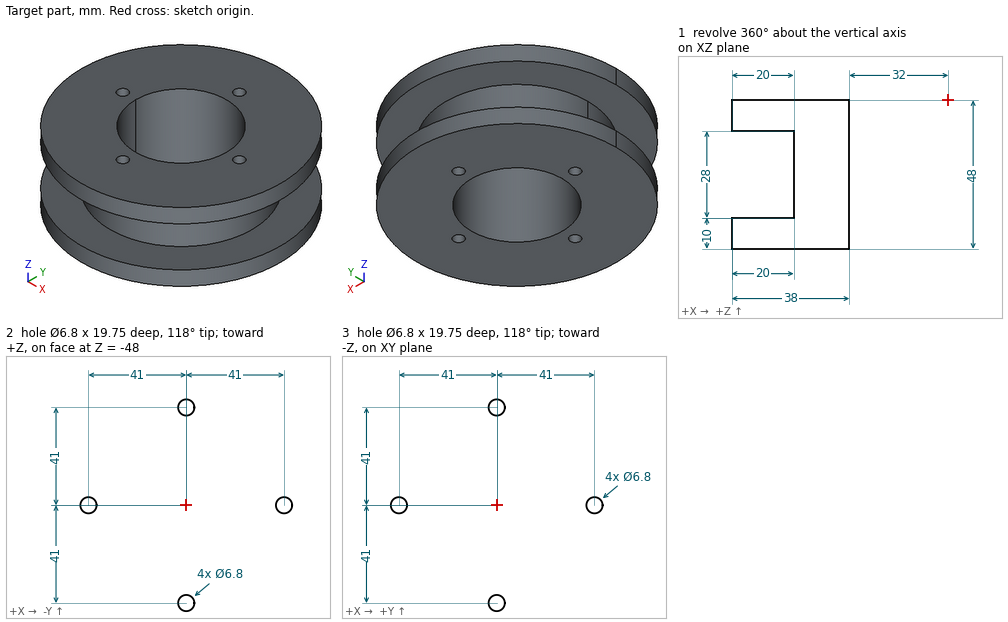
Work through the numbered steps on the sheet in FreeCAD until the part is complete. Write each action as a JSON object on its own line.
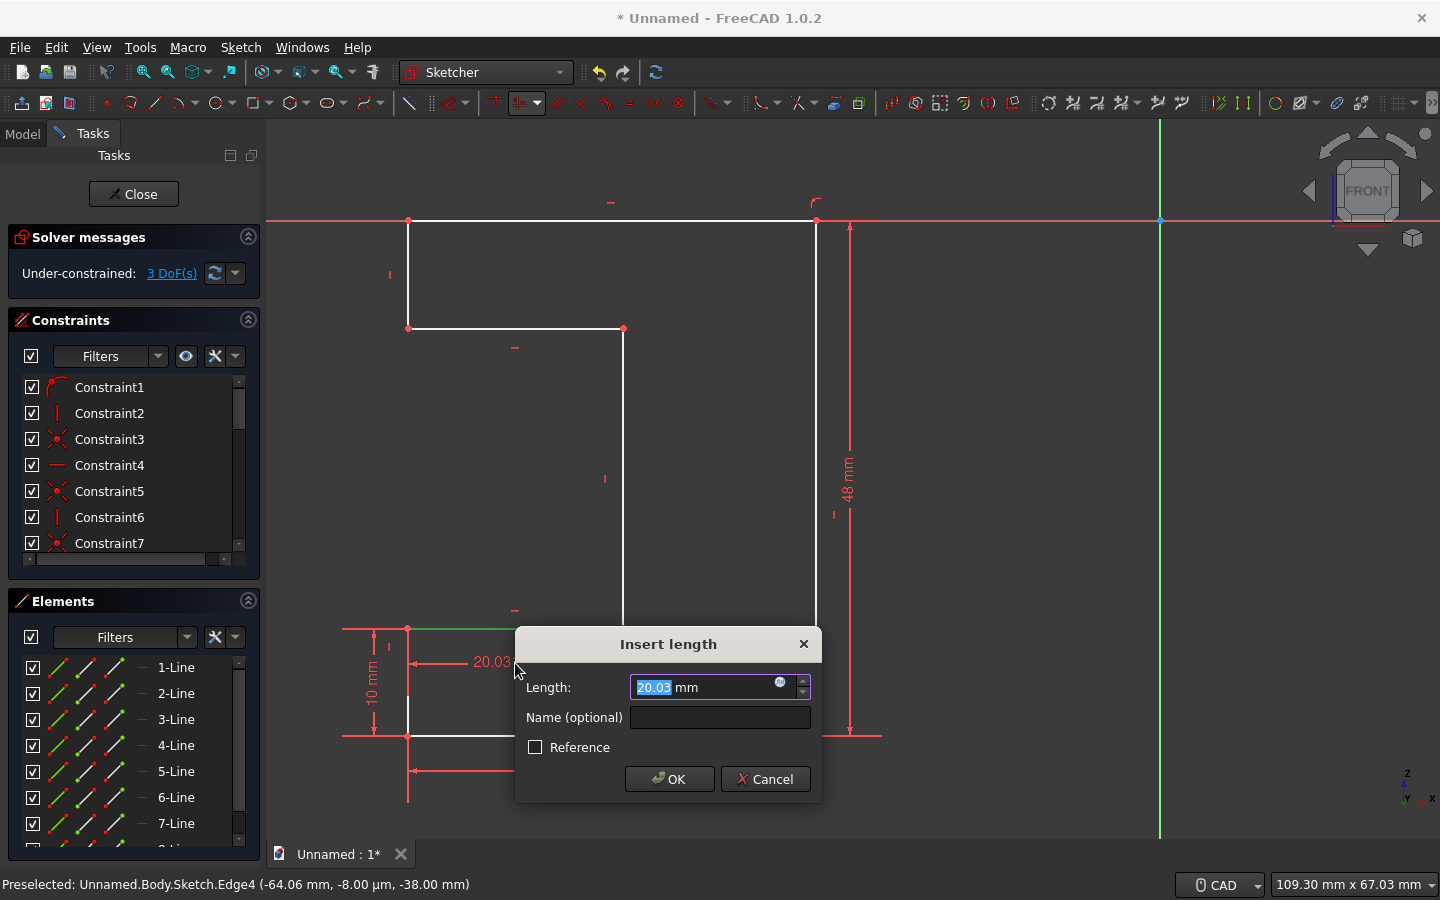
{"action": "type", "text": "20"}
{"action": "key", "text": "Return"}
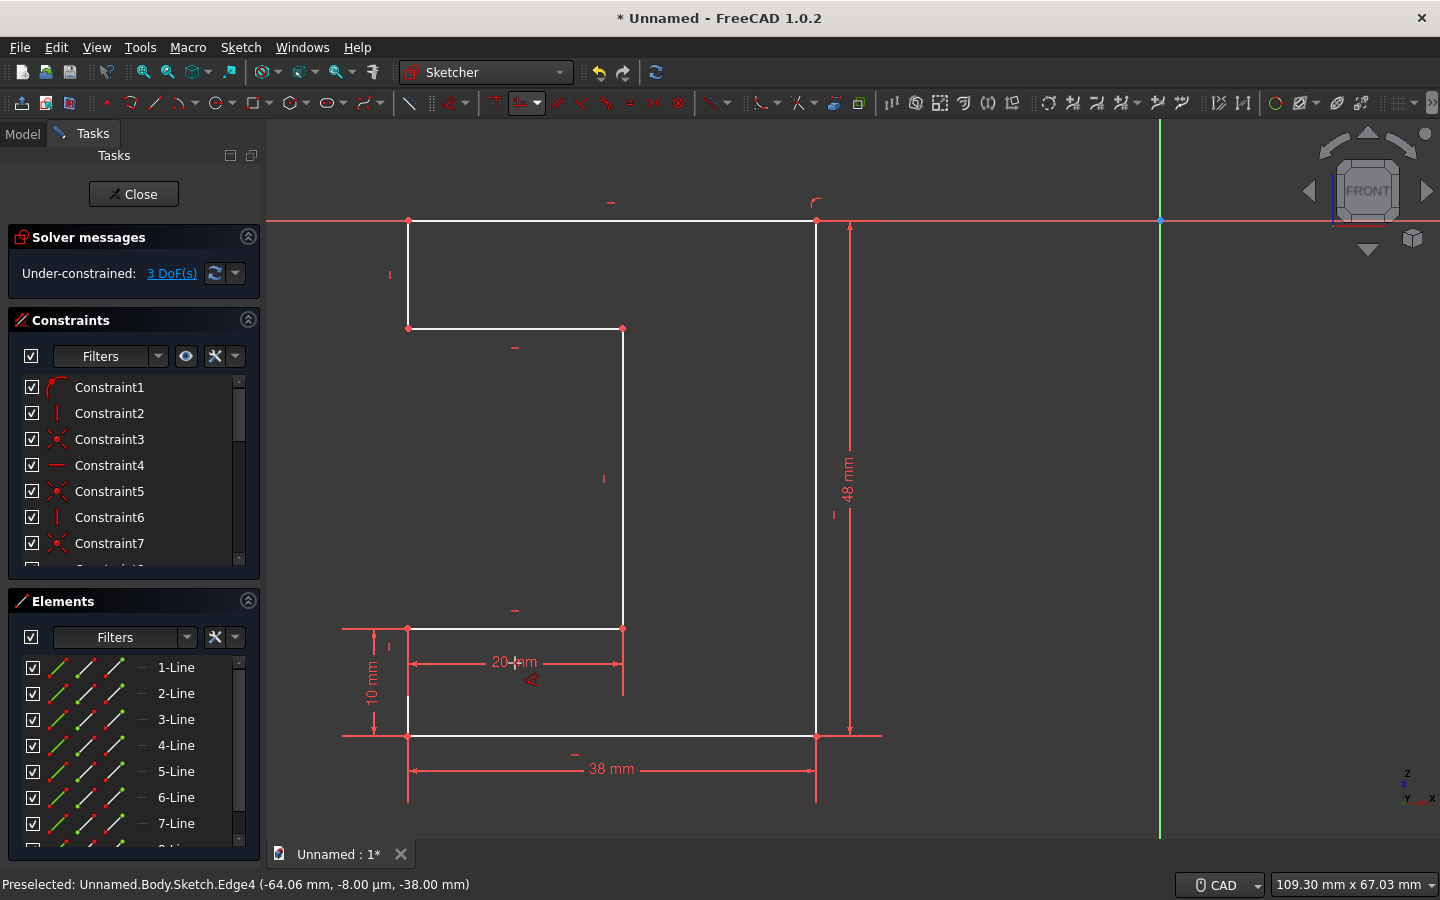
{"action": "left_click", "coordinate": [623, 539]}
{"action": "left_click", "coordinate": [589, 479]}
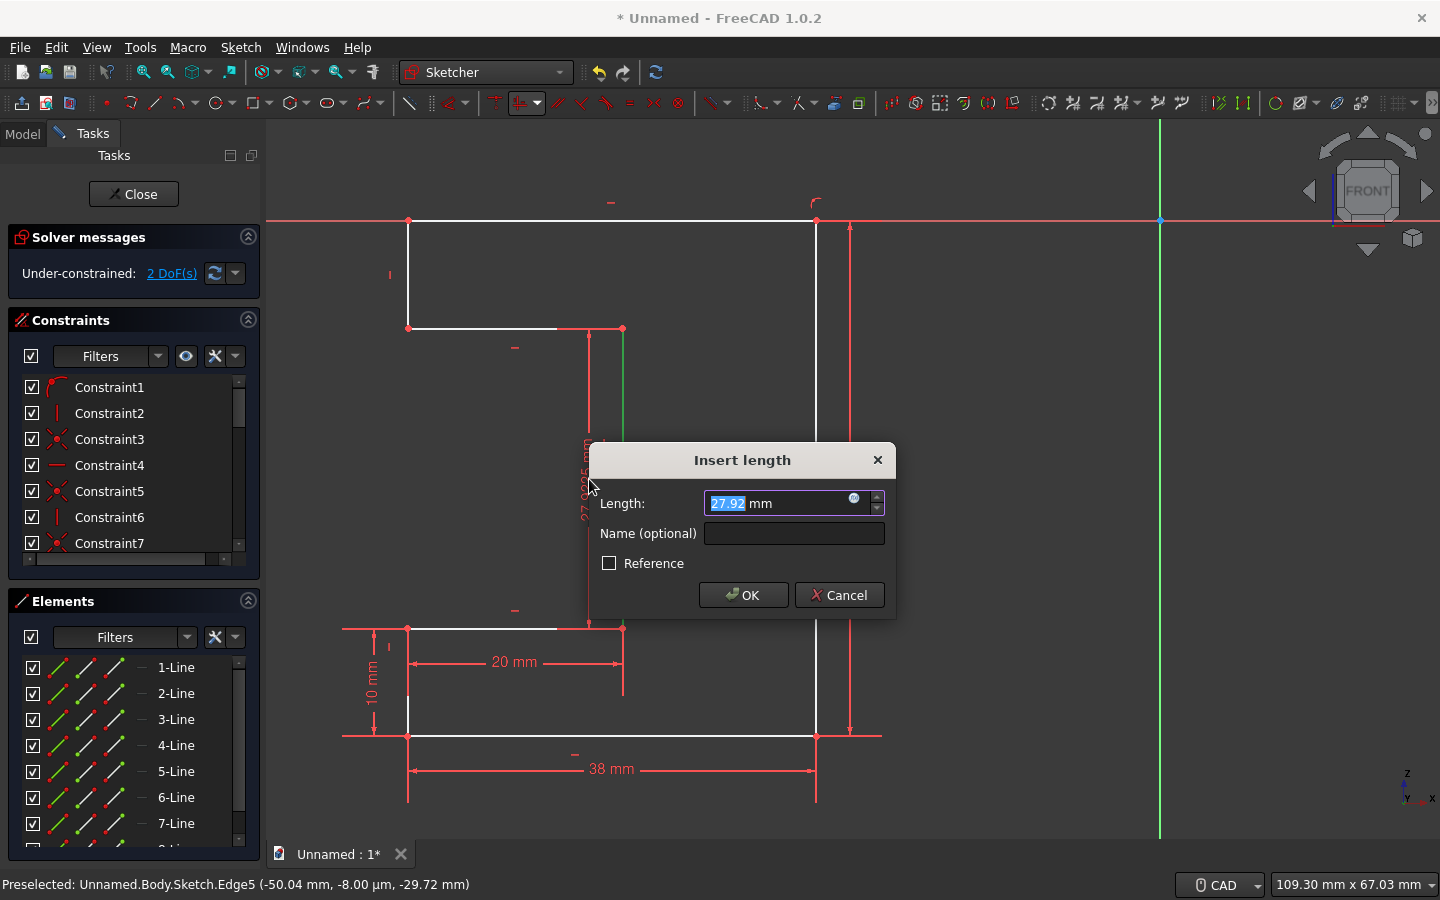
{"action": "type", "text": "28"}
{"action": "key", "text": "Return"}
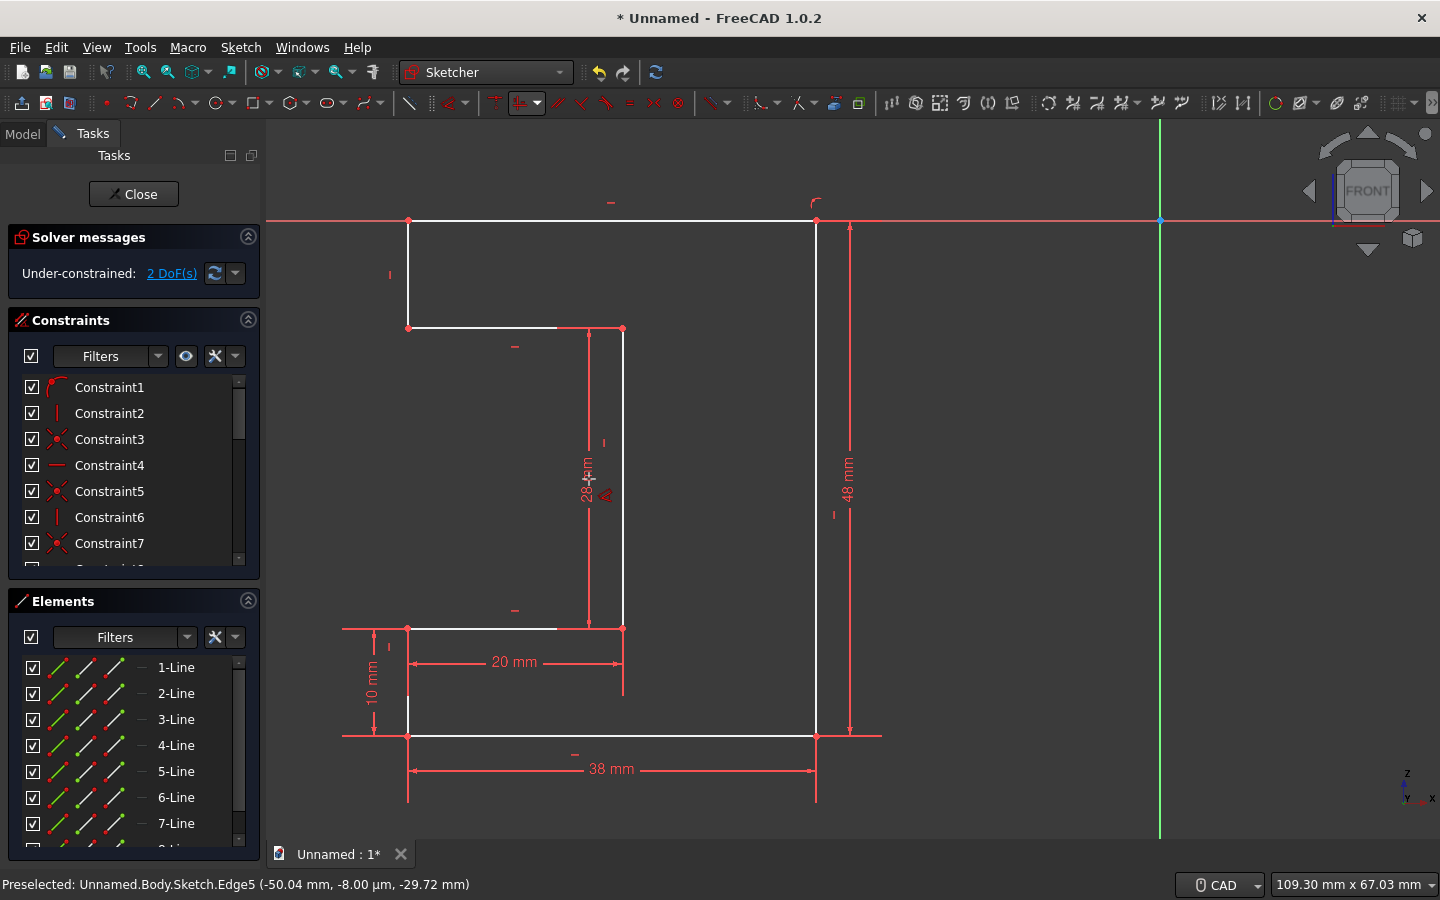
{"action": "left_click", "coordinate": [558, 328]}
{"action": "left_click", "coordinate": [515, 294]}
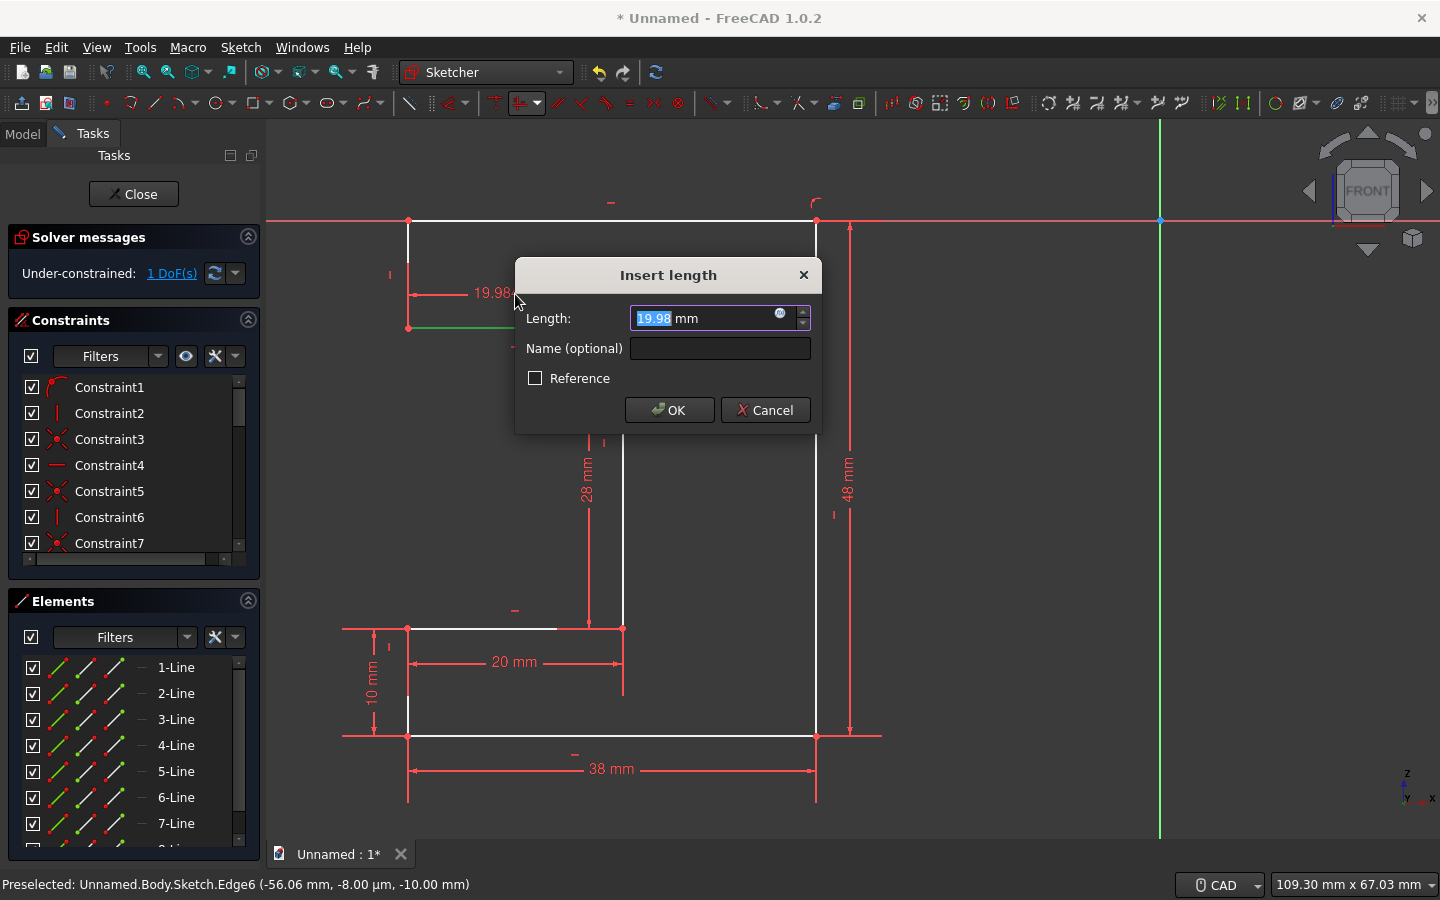
{"action": "type", "text": "20"}
{"action": "key", "text": "Return"}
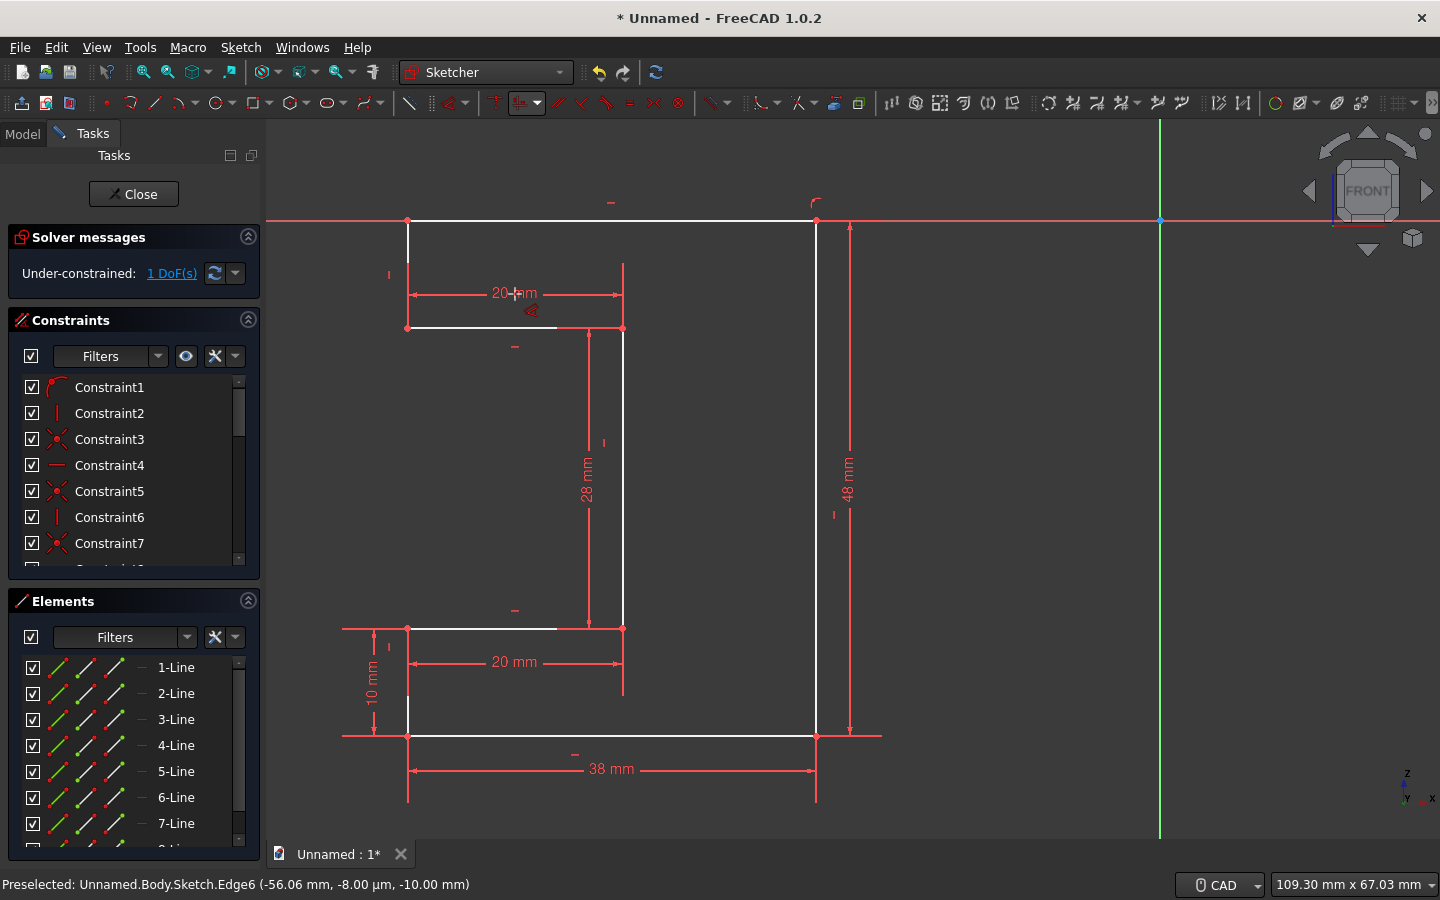
{"action": "left_click", "coordinate": [816, 221]}
{"action": "left_click", "coordinate": [988, 187]}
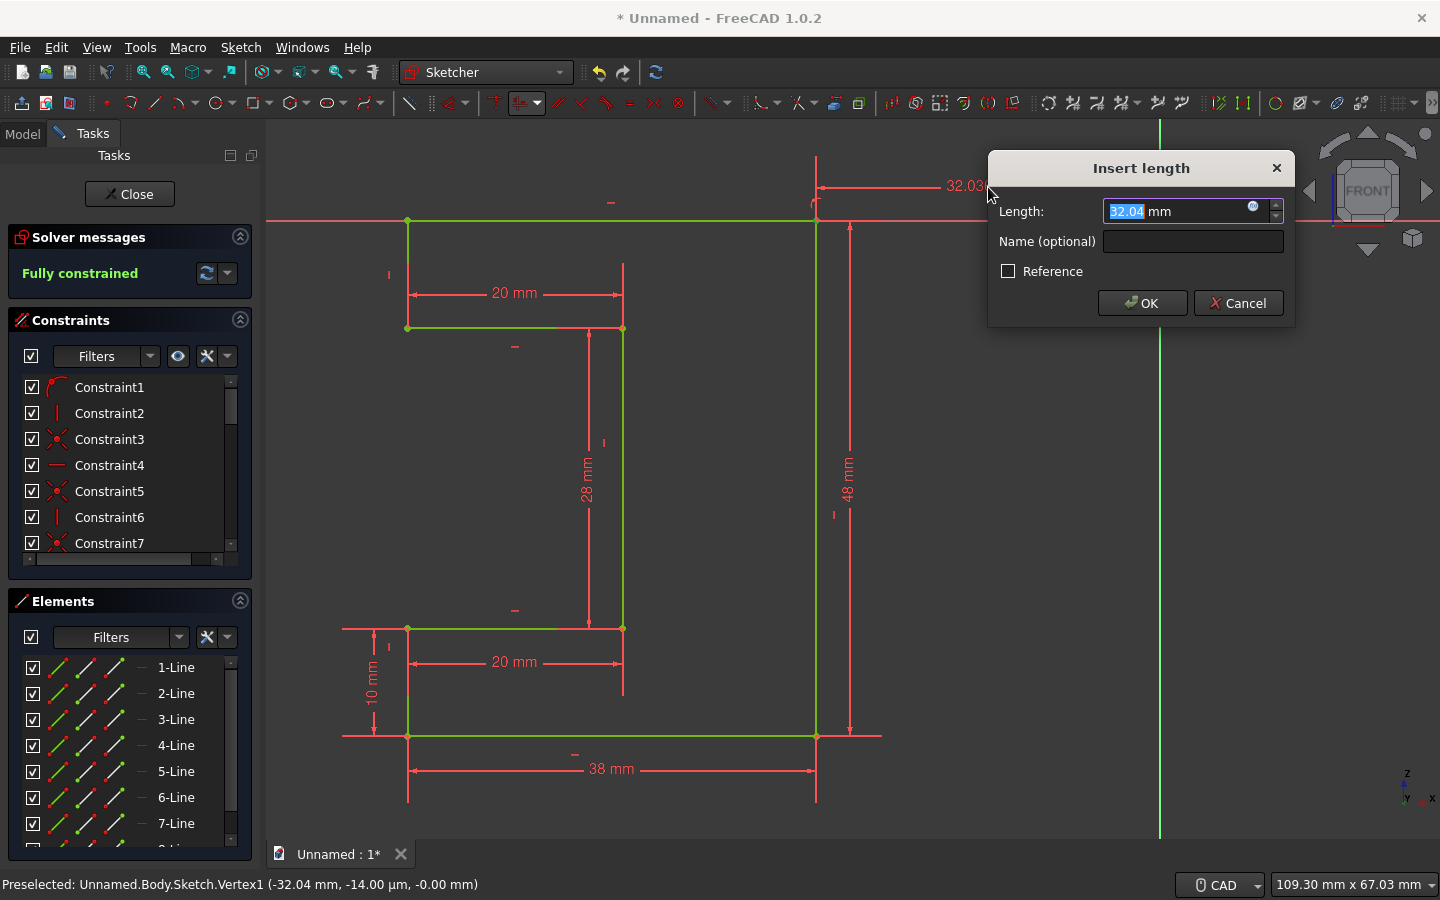
{"action": "type", "text": "32"}
{"action": "key", "text": "Return"}
{"action": "key", "text": "Escape"}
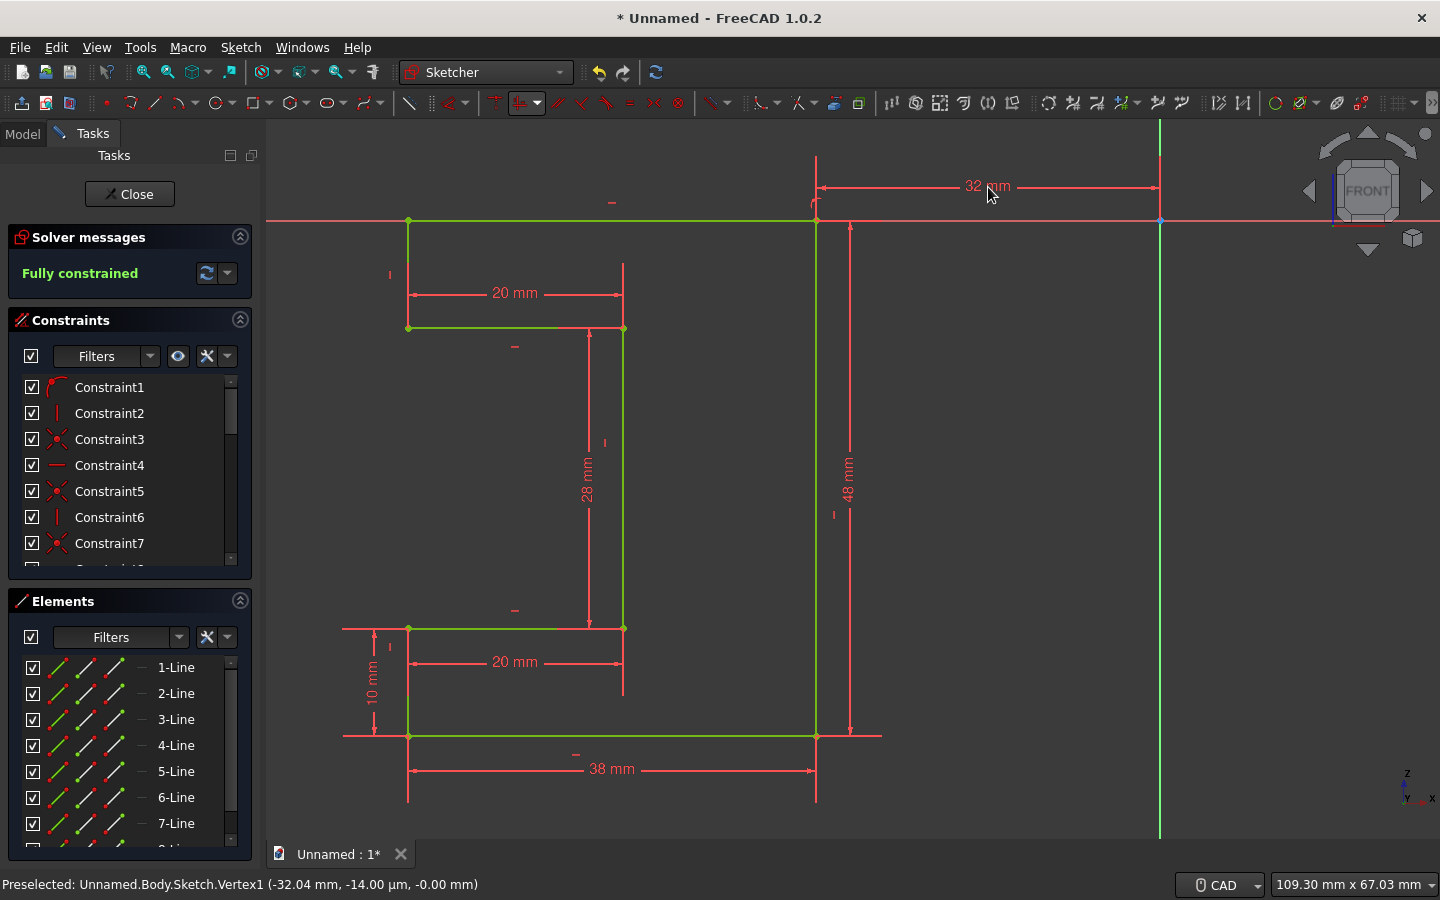
{"action": "left_click", "coordinate": [130, 194]}